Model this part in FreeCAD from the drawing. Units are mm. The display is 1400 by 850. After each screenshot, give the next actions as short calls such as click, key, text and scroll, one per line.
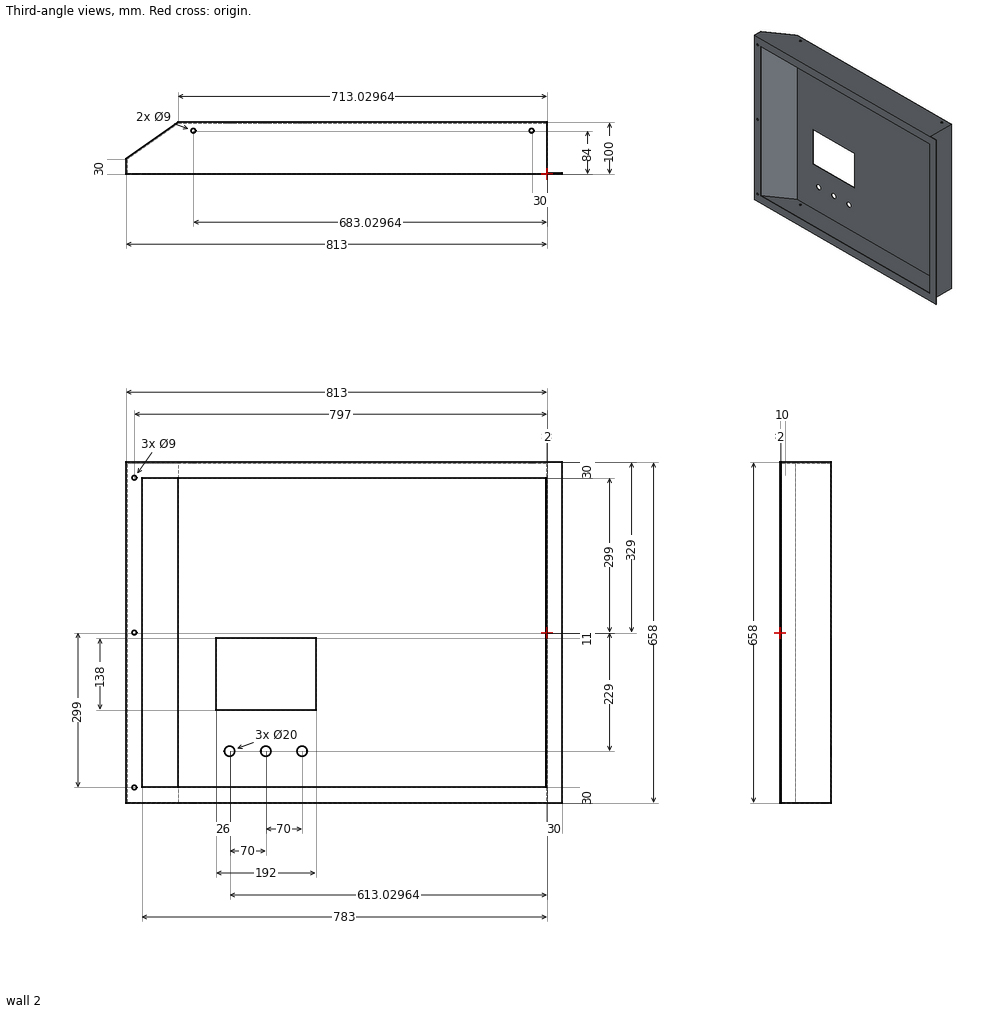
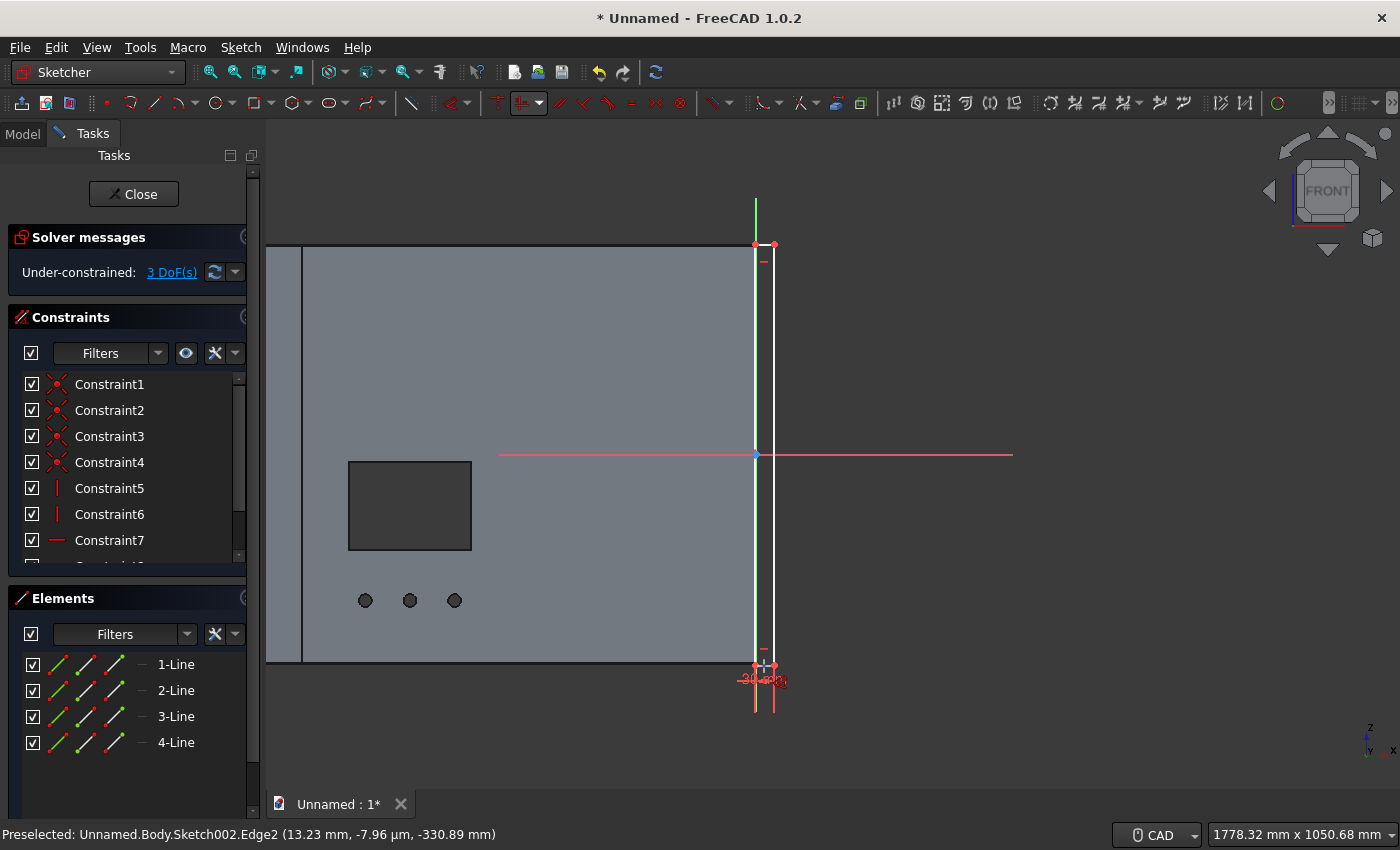
scroll(755, 245, up, 18)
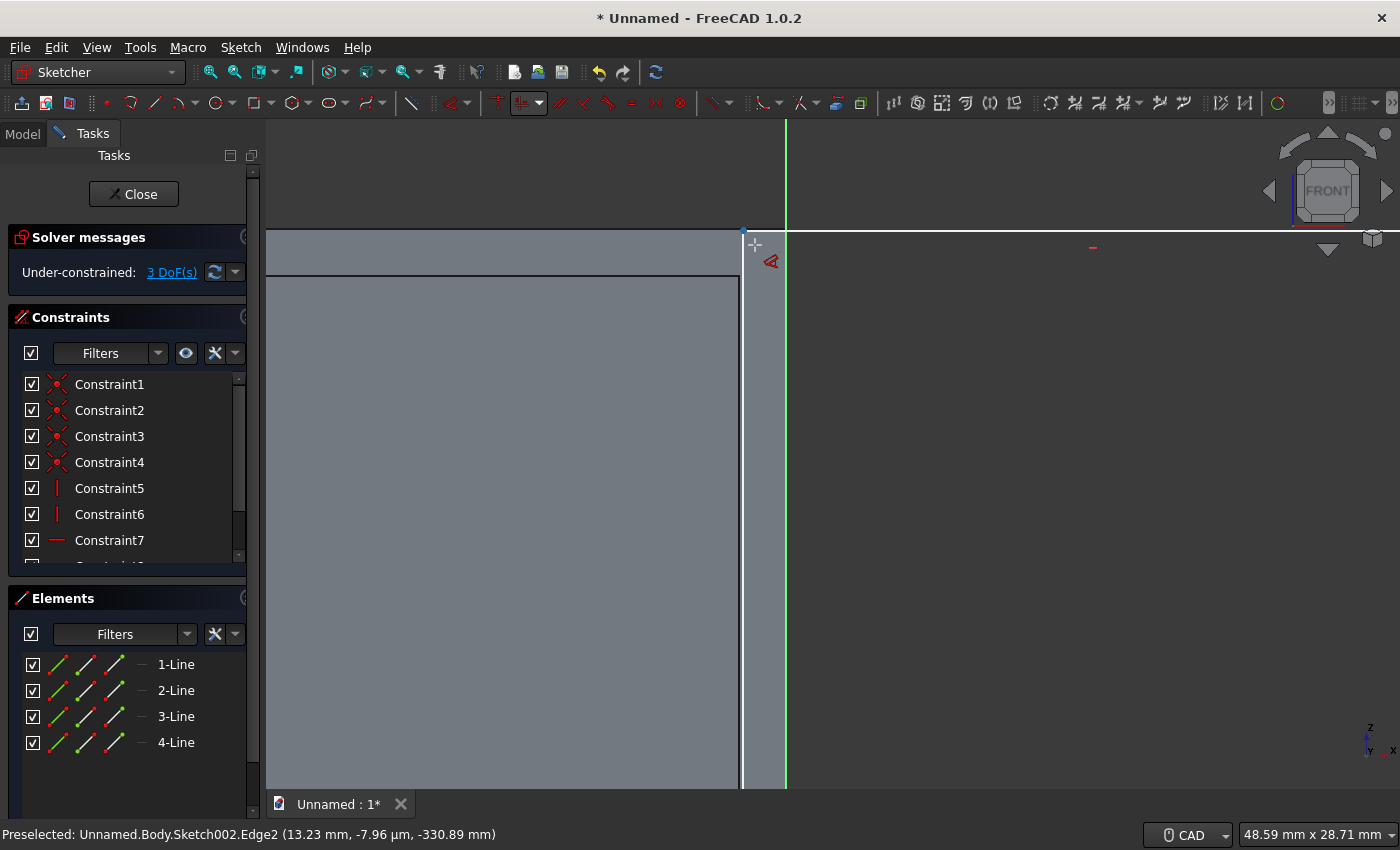
click(743, 231)
click(765, 197)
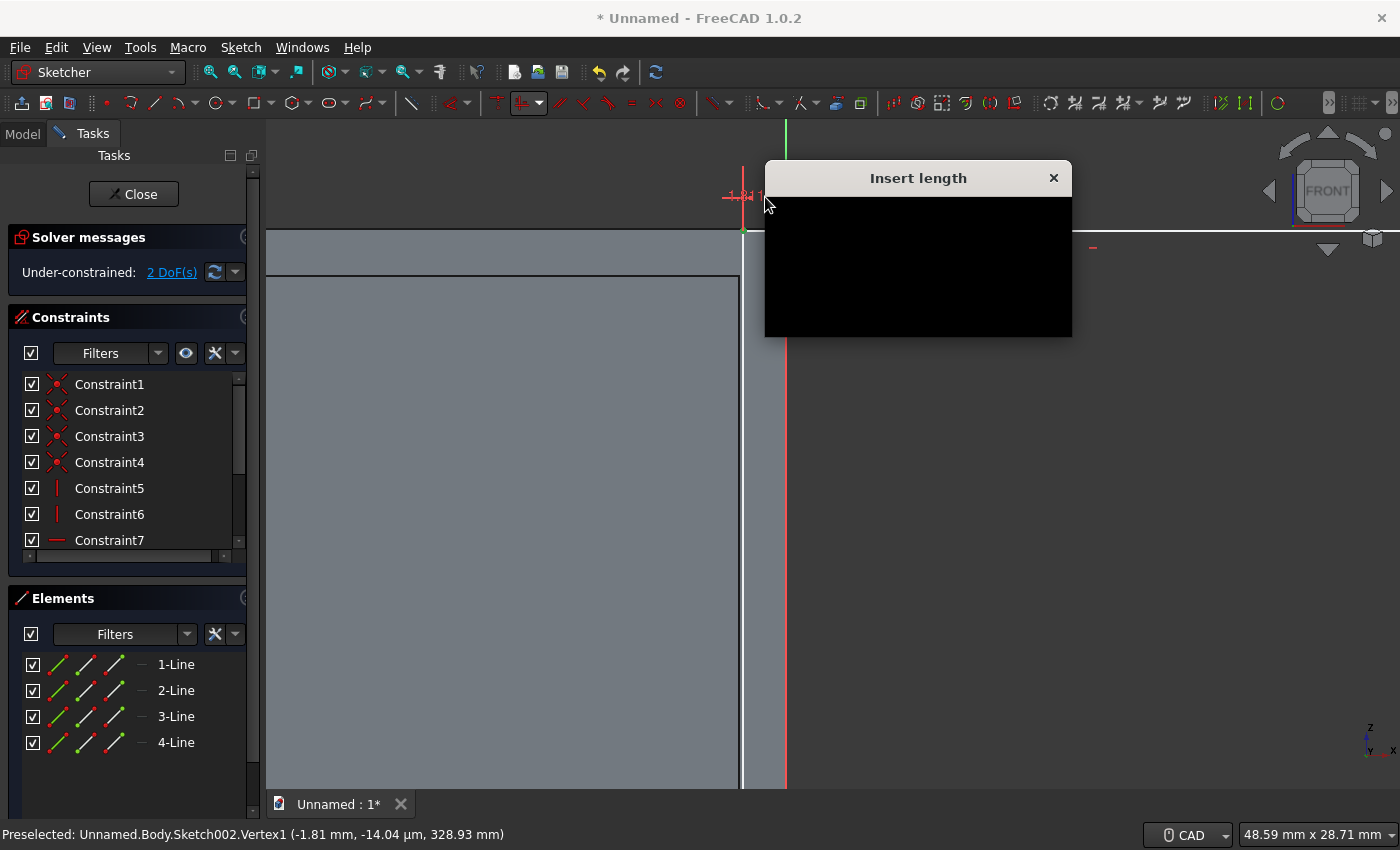
text(2)
key(Return)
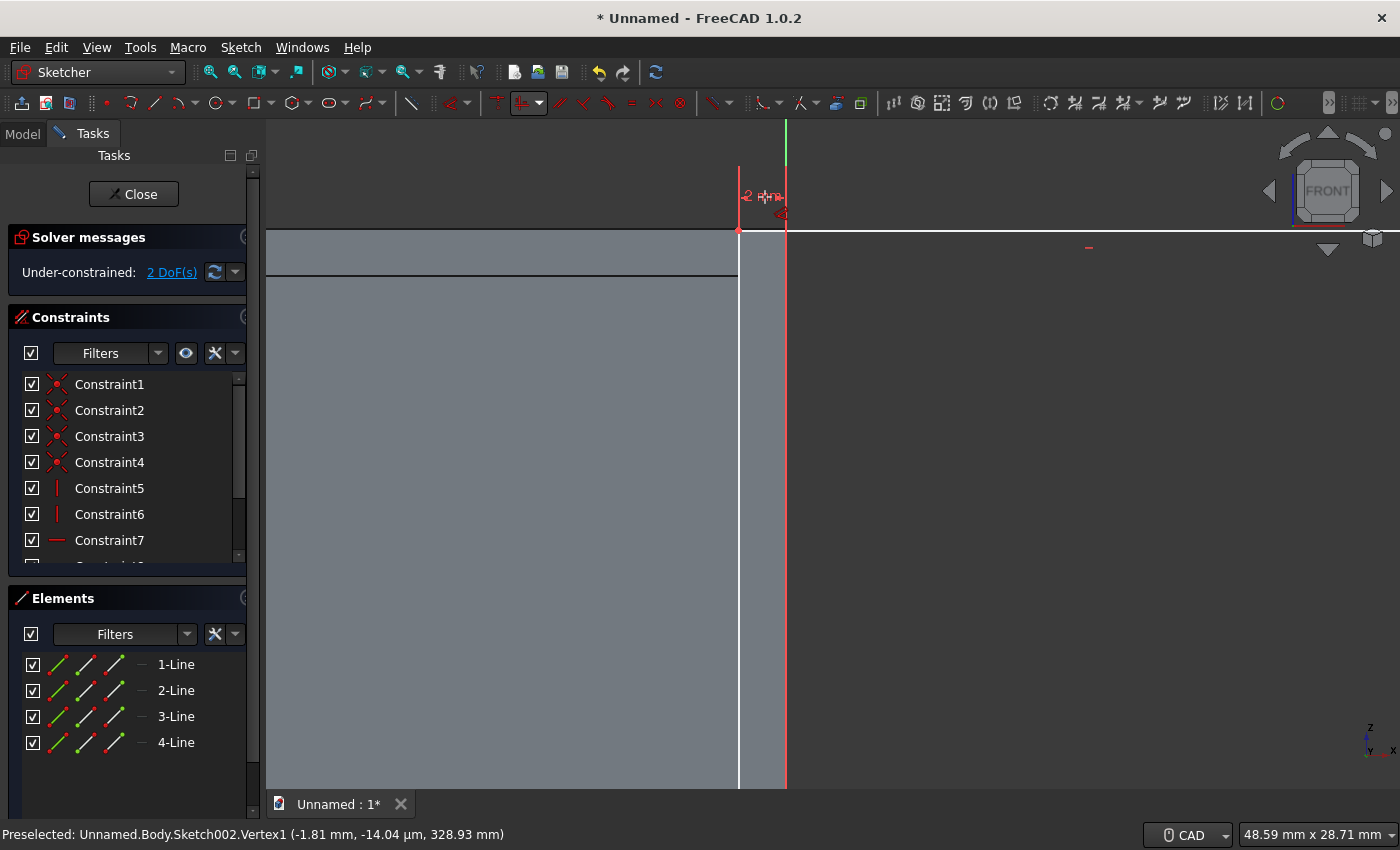
scroll(753, 197, down, 17)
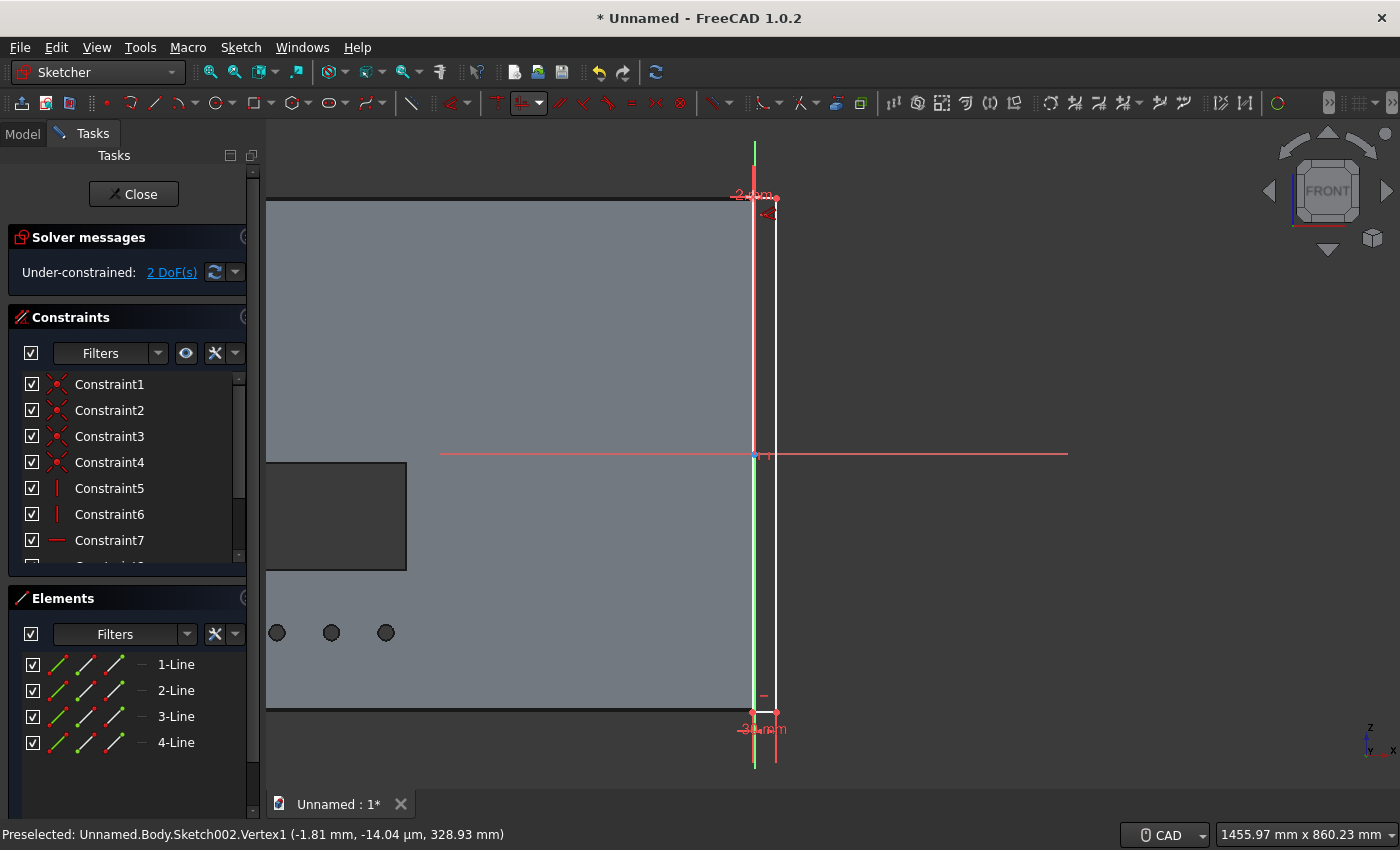
scroll(753, 352, up, 11)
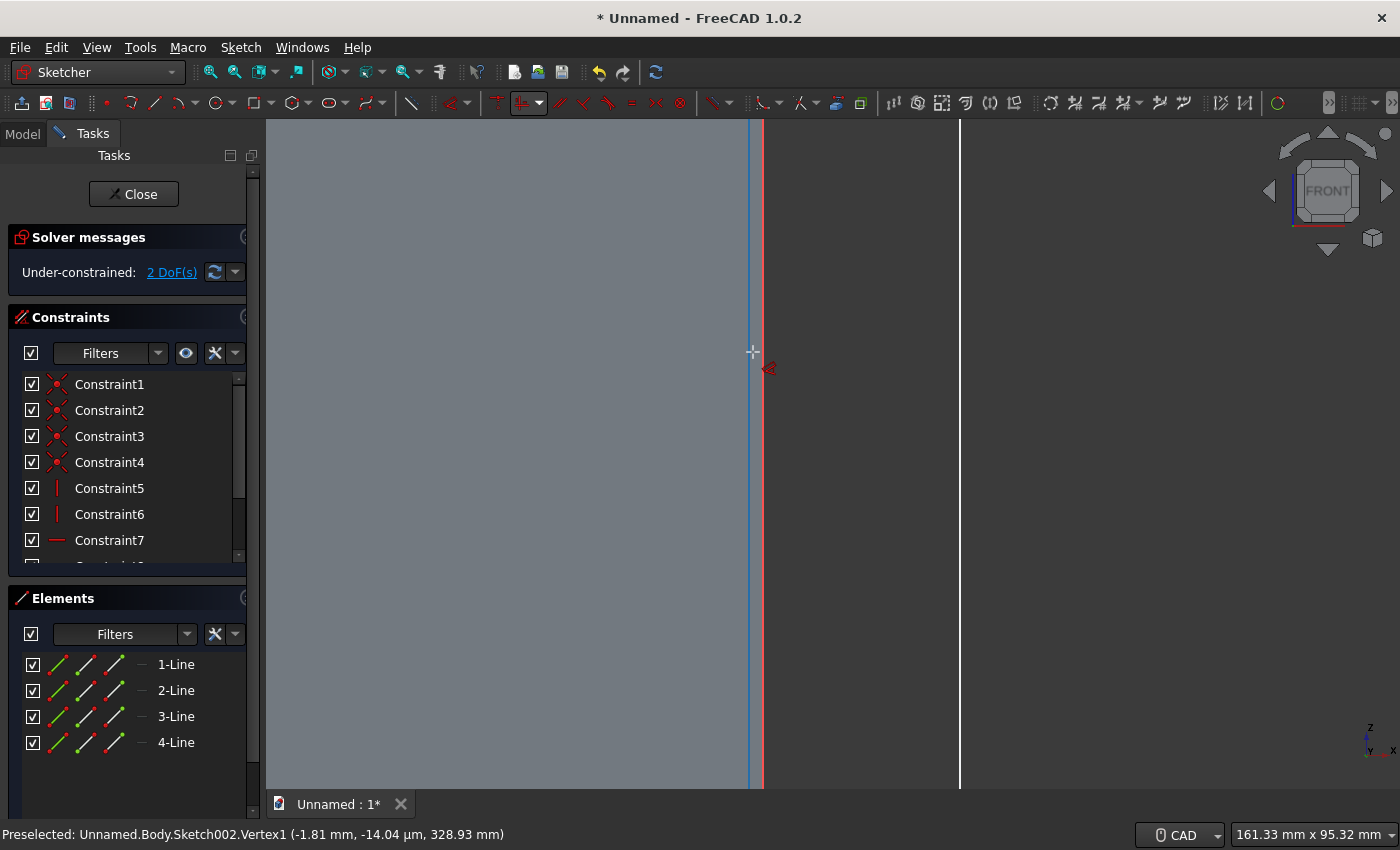
click(749, 353)
click(715, 454)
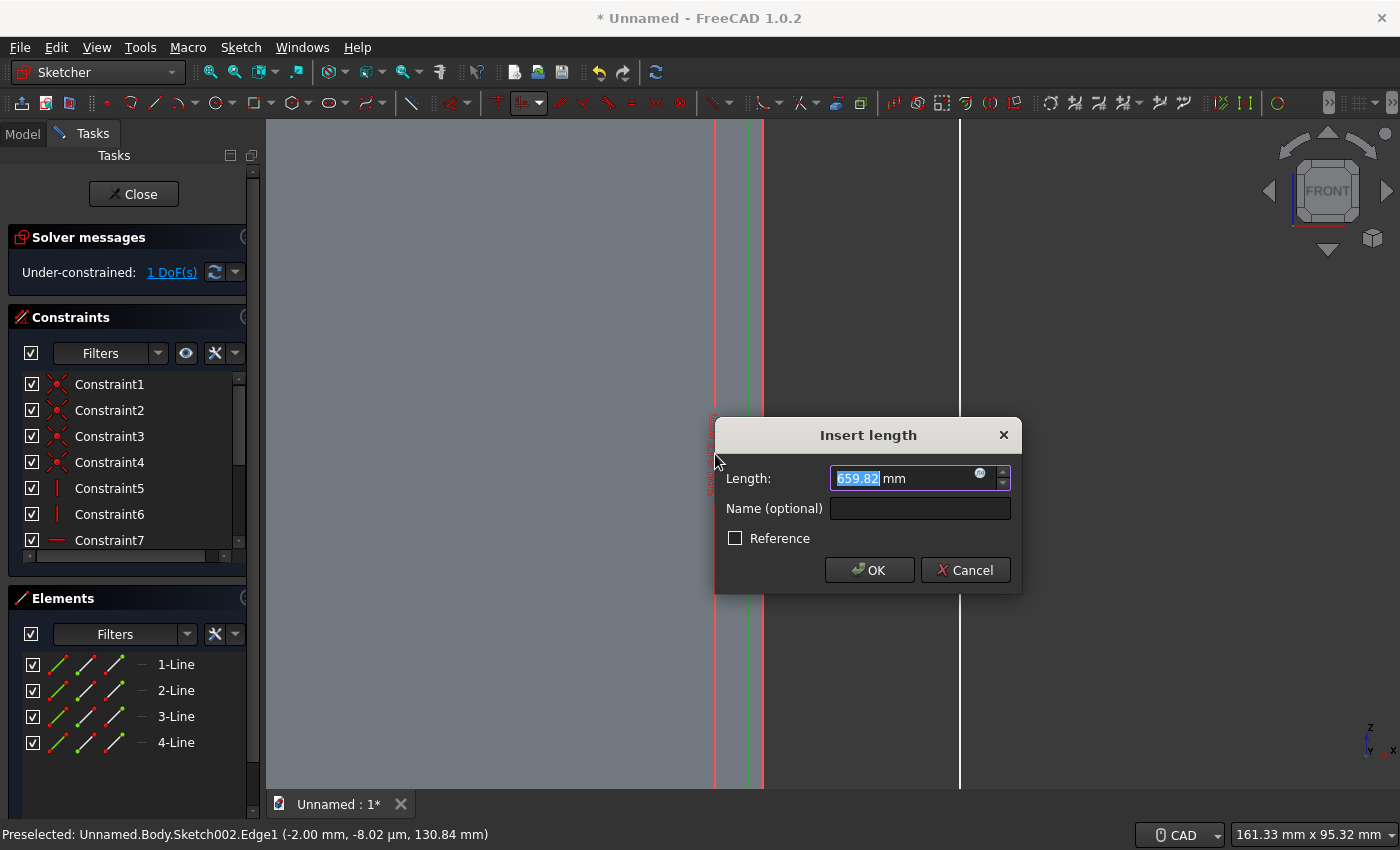
text(658)
key(Return)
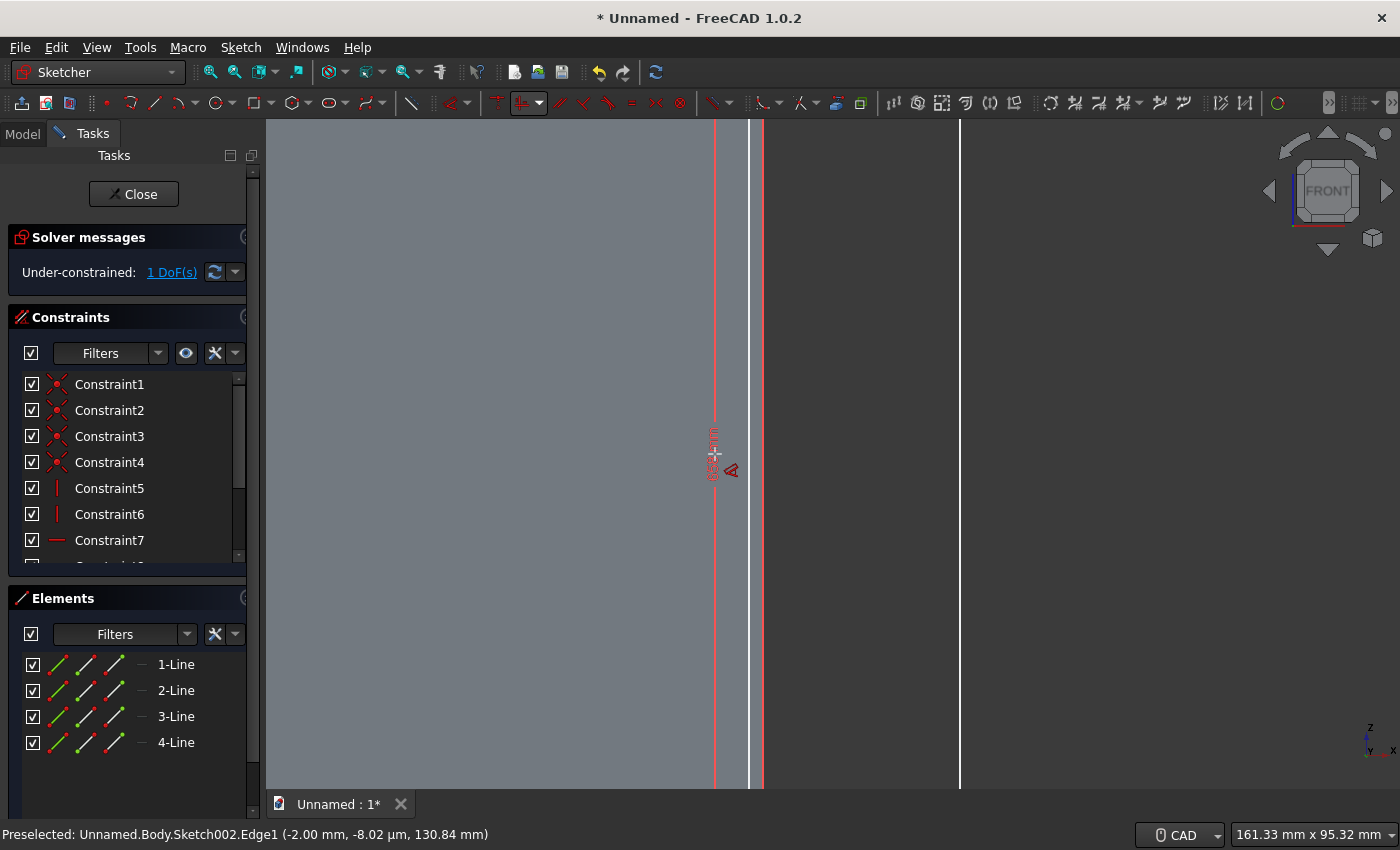
scroll(756, 372, down, 12)